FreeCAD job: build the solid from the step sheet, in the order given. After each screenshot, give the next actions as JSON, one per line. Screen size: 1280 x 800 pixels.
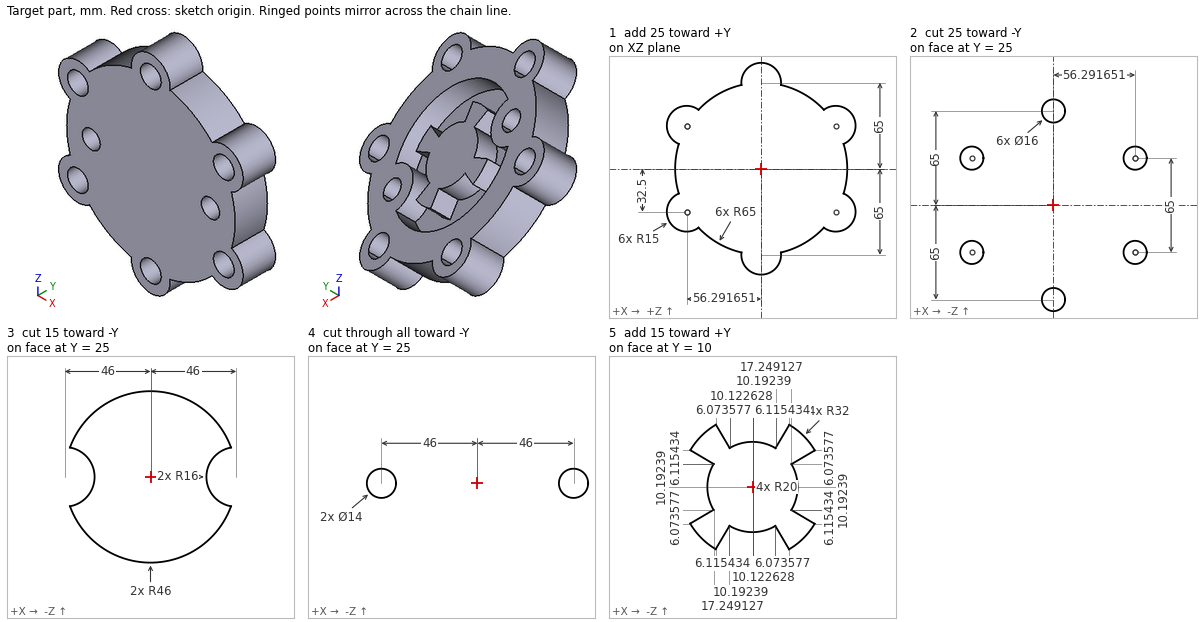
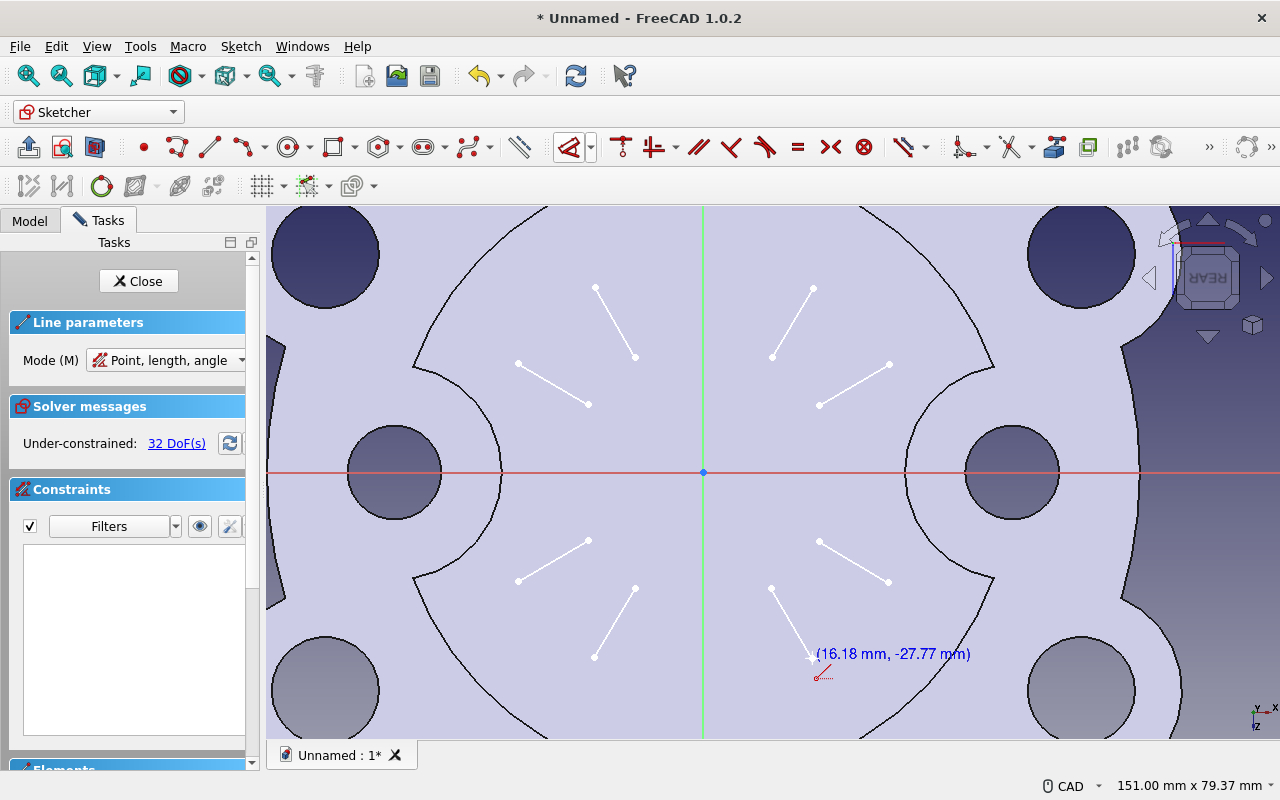
{"action": "key", "text": "g 3 a"}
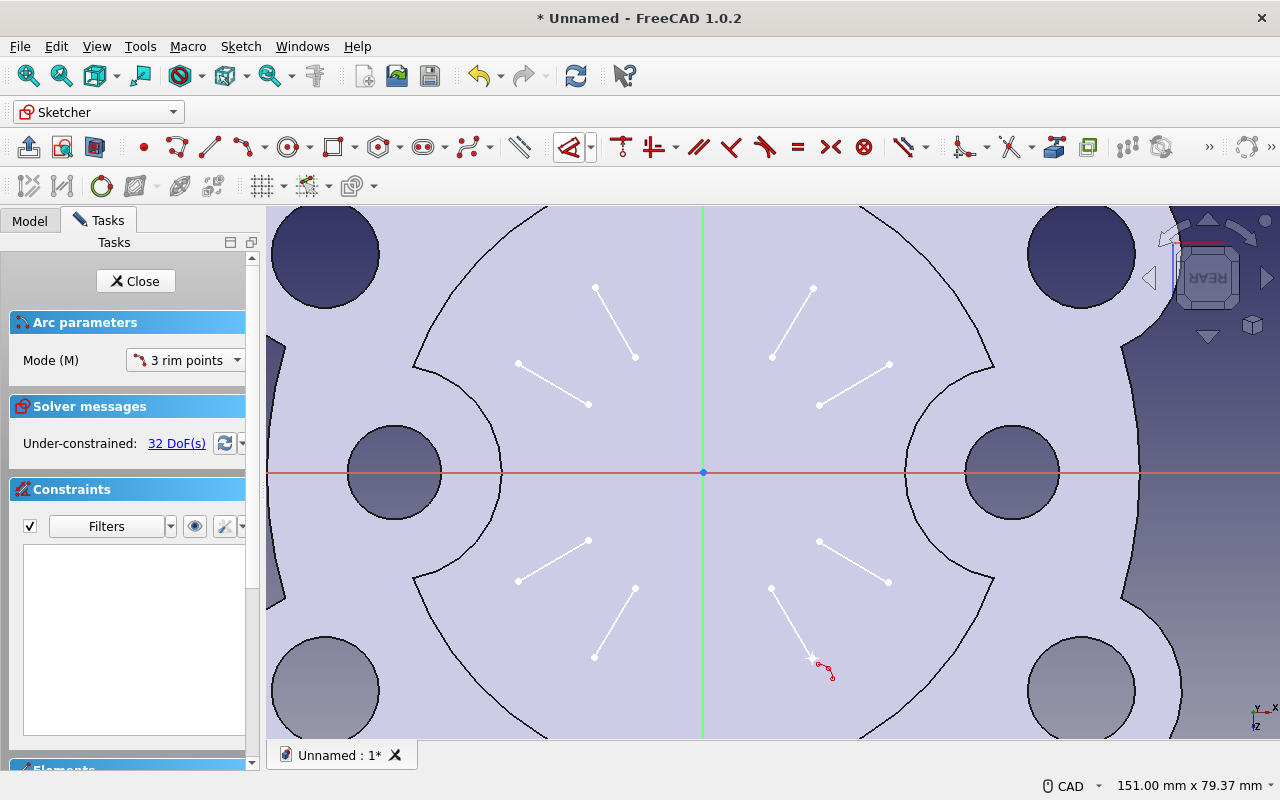
{"action": "left_click", "coordinate": [819, 542]}
{"action": "left_click", "coordinate": [819, 406]}
{"action": "left_click", "coordinate": [837, 487]}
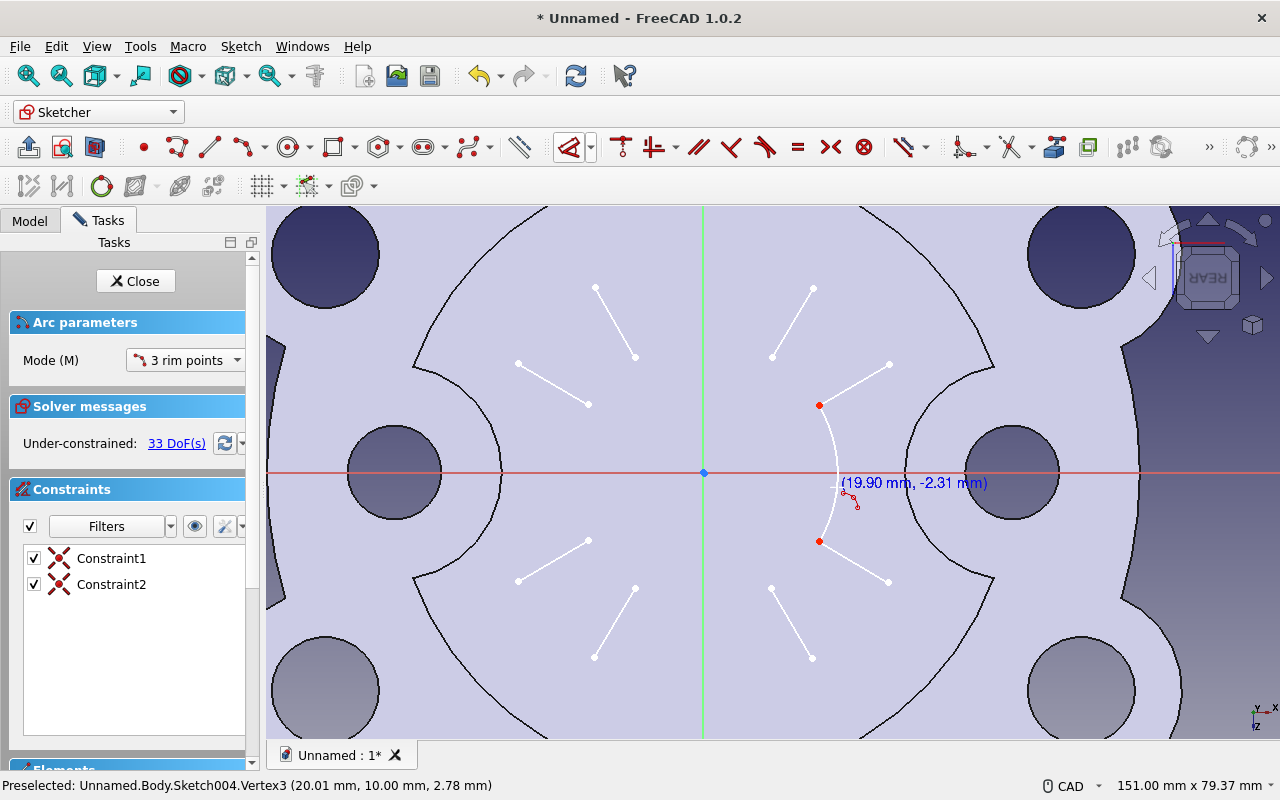
{"action": "left_click", "coordinate": [889, 365]}
{"action": "left_click", "coordinate": [813, 289]}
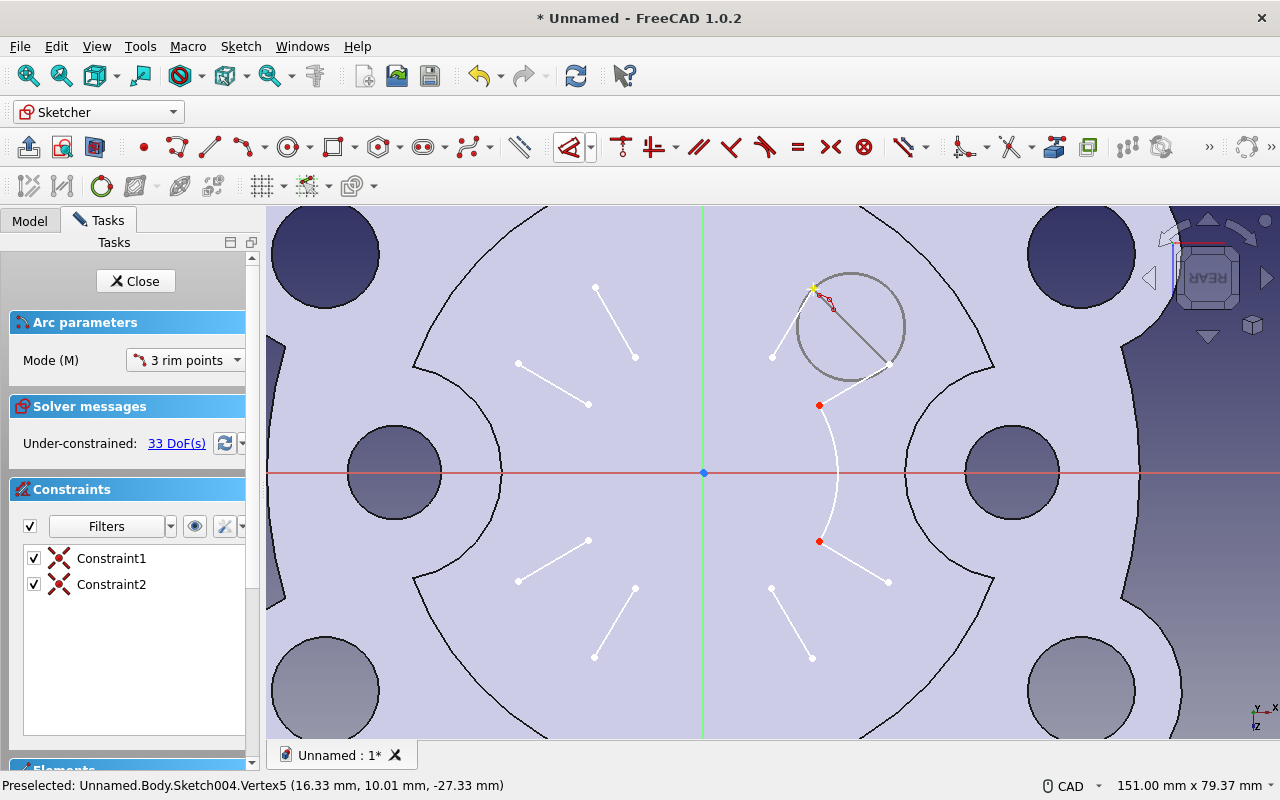
{"action": "scroll", "coordinate": [856, 321], "scroll_direction": "up", "scroll_amount": 5}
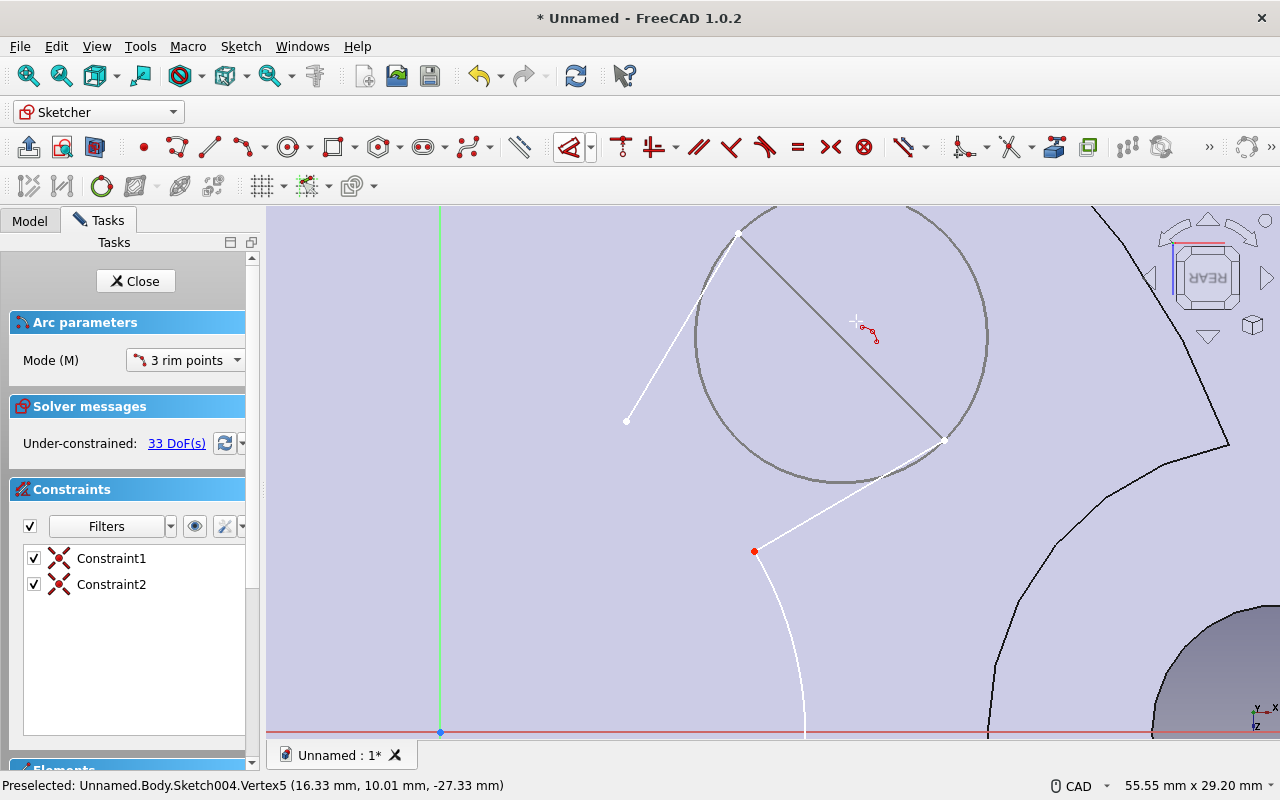
{"action": "left_click", "coordinate": [854, 320]}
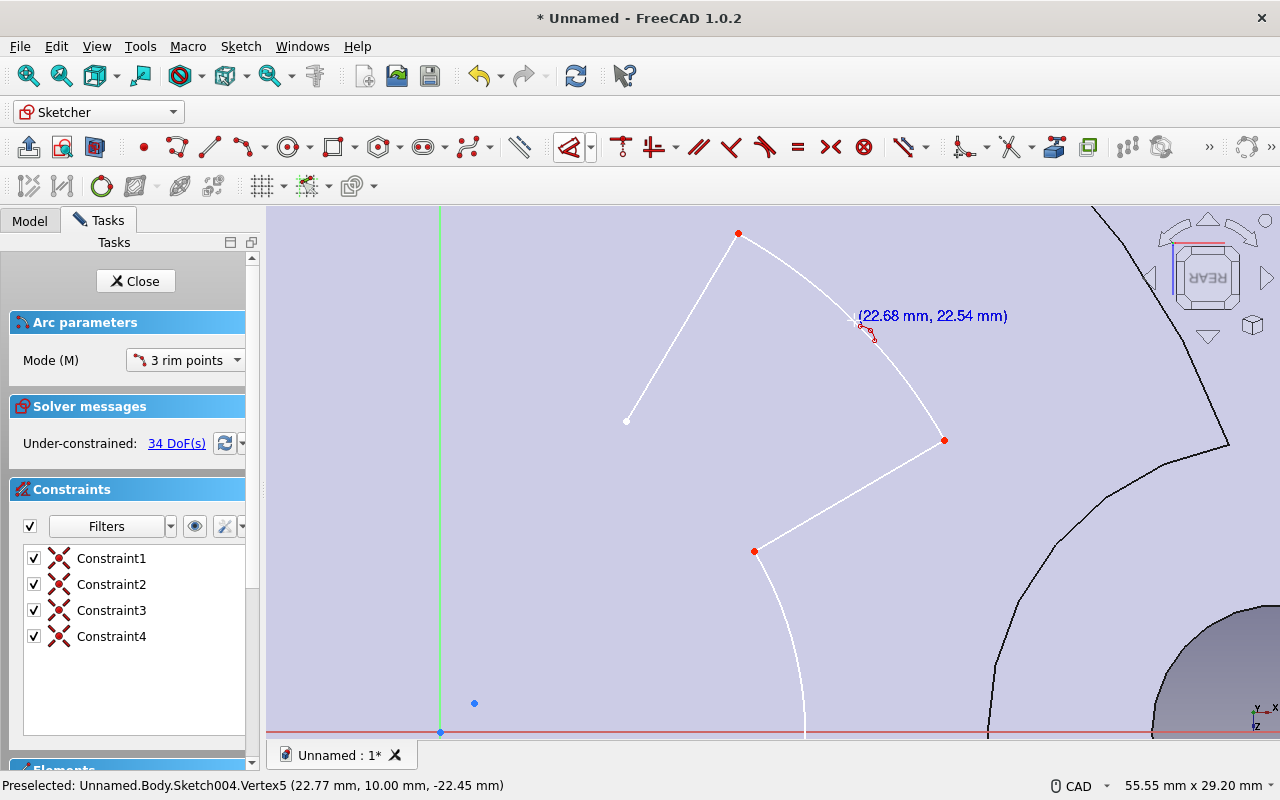
{"action": "left_click", "coordinate": [627, 421]}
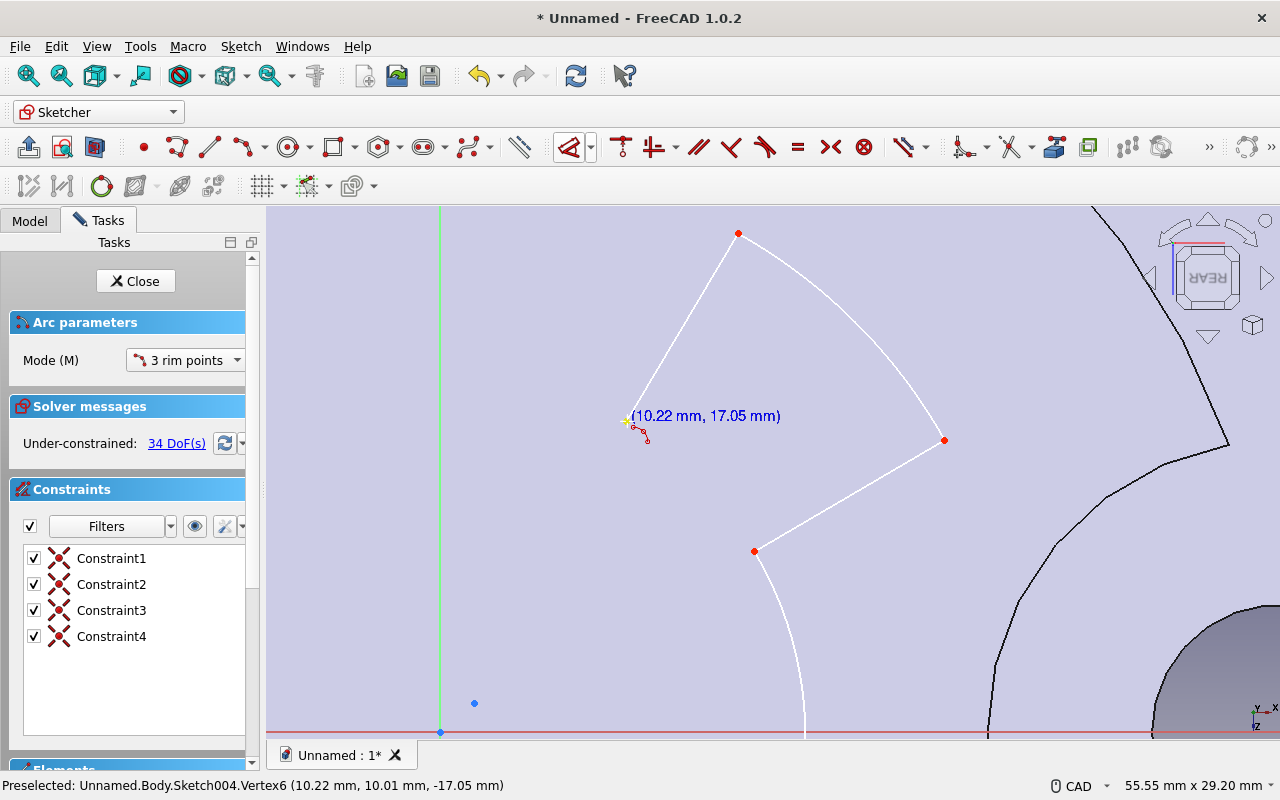
{"action": "scroll", "coordinate": [858, 321], "scroll_direction": "down", "scroll_amount": 5}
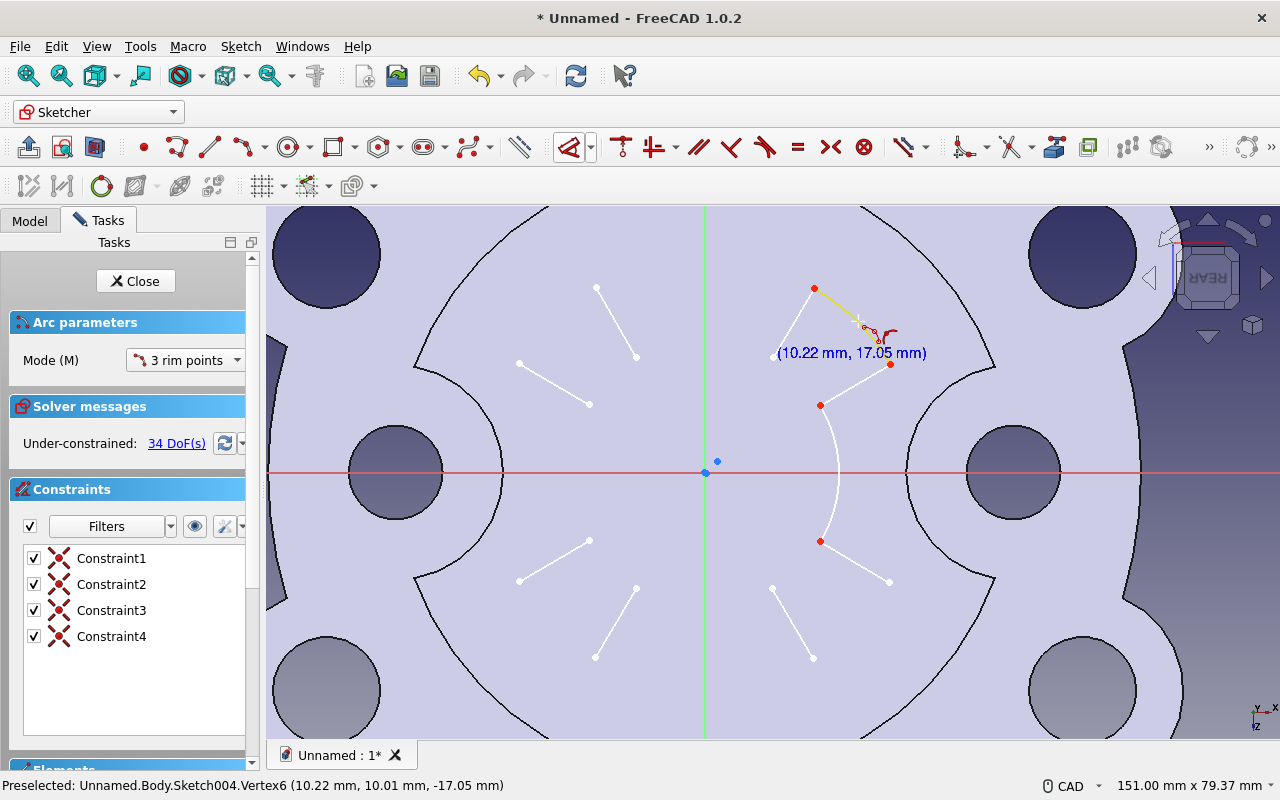
{"action": "left_click", "coordinate": [636, 358]}
{"action": "left_click", "coordinate": [719, 339]}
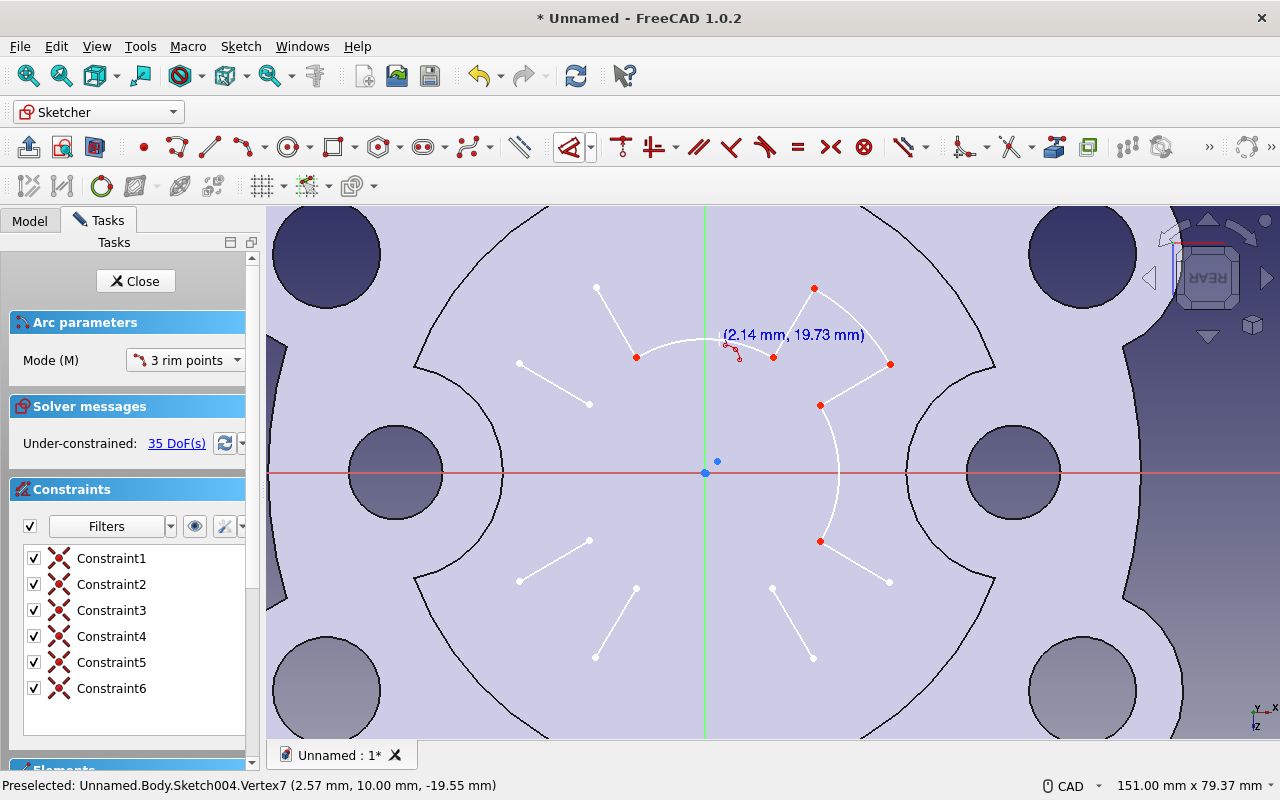
{"action": "left_click", "coordinate": [596, 288]}
{"action": "left_click", "coordinate": [519, 364]}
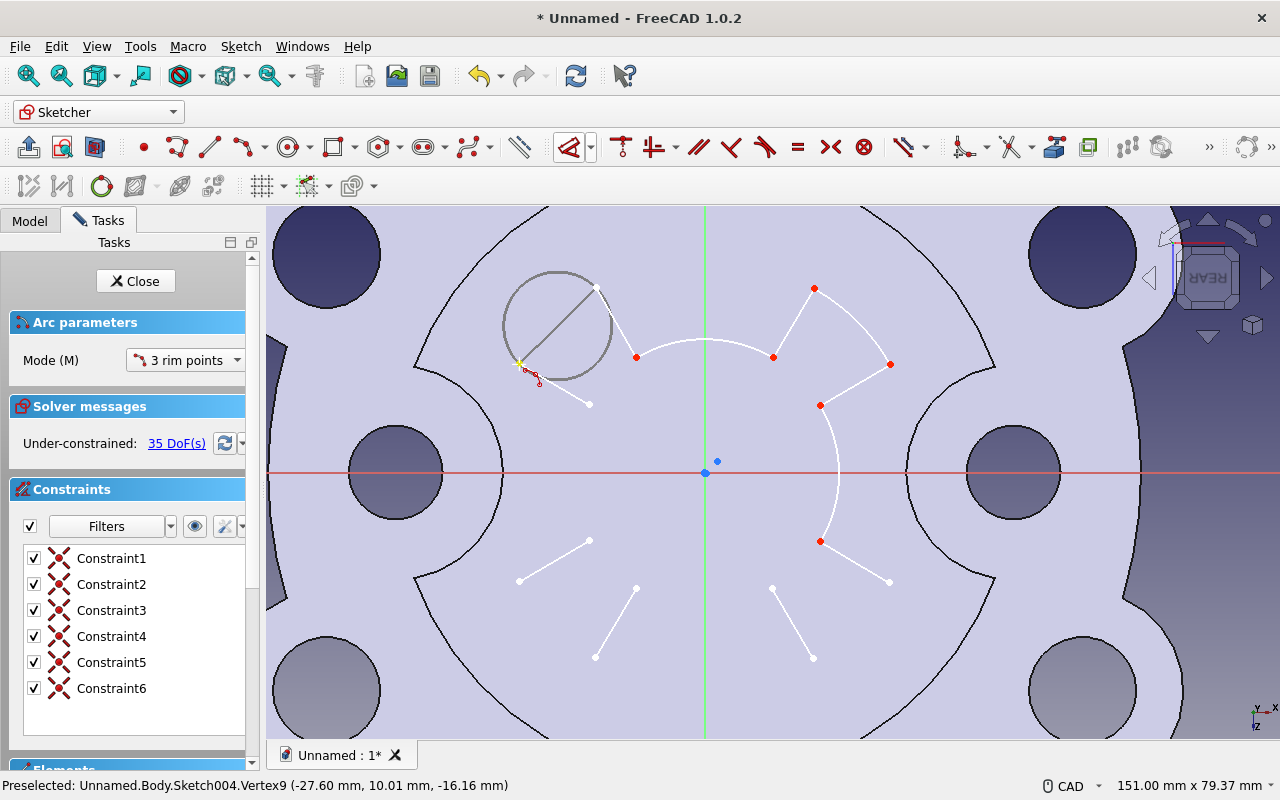
{"action": "scroll", "coordinate": [553, 320], "scroll_direction": "up", "scroll_amount": 5}